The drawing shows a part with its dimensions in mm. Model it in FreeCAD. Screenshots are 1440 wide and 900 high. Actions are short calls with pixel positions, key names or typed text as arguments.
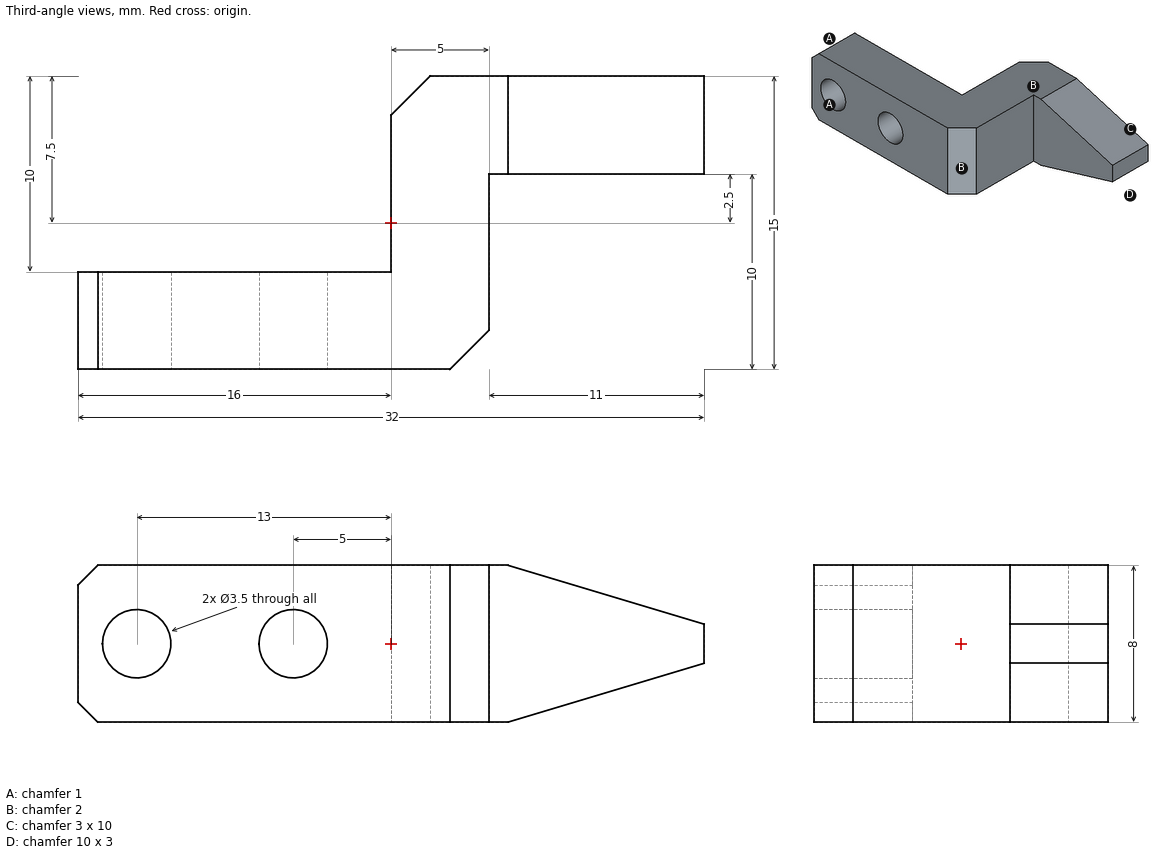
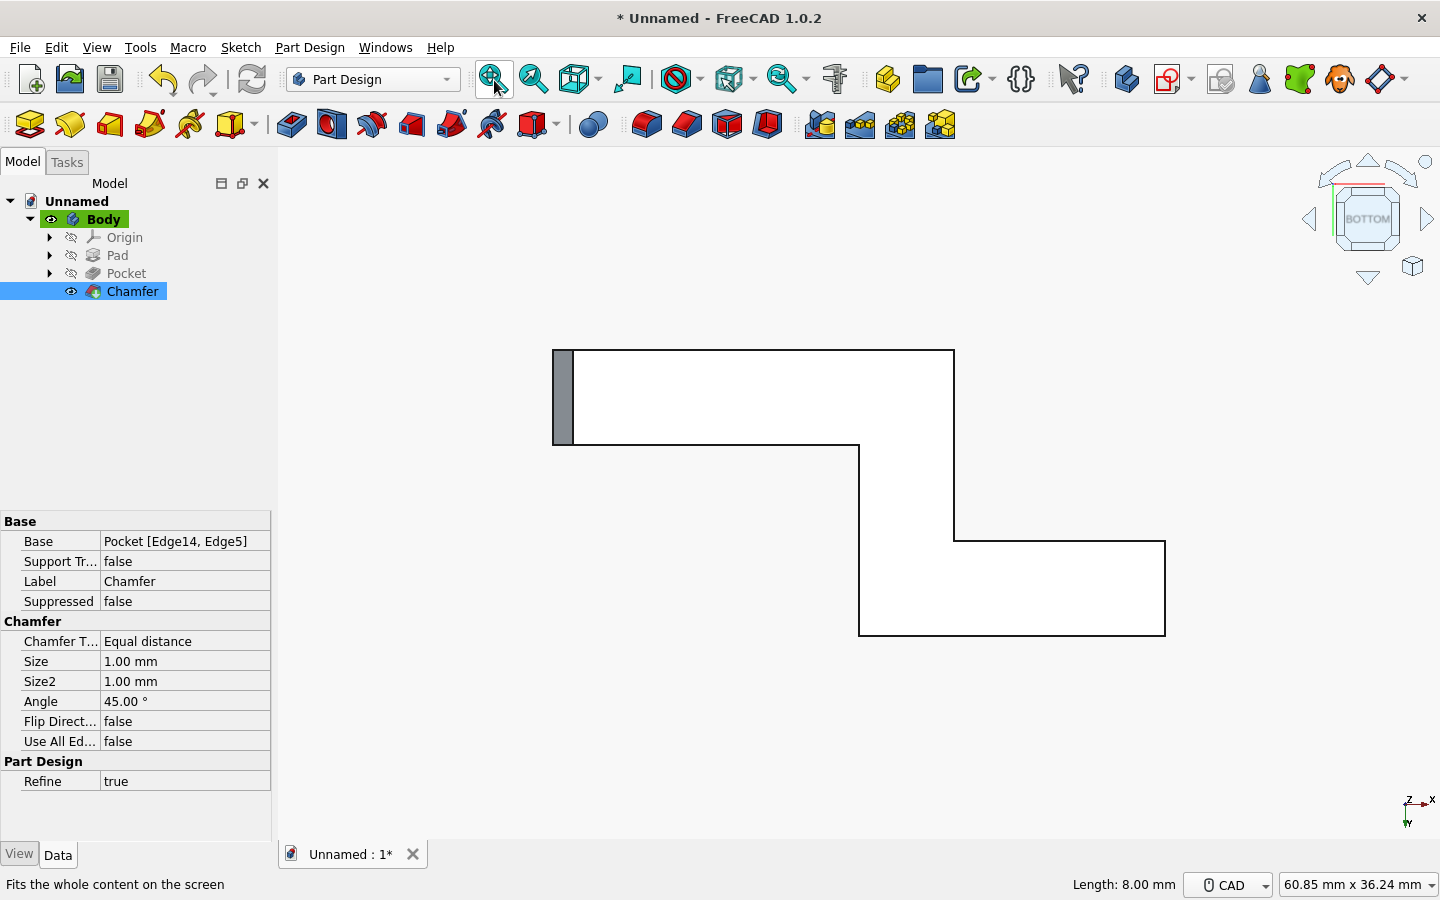
key(4)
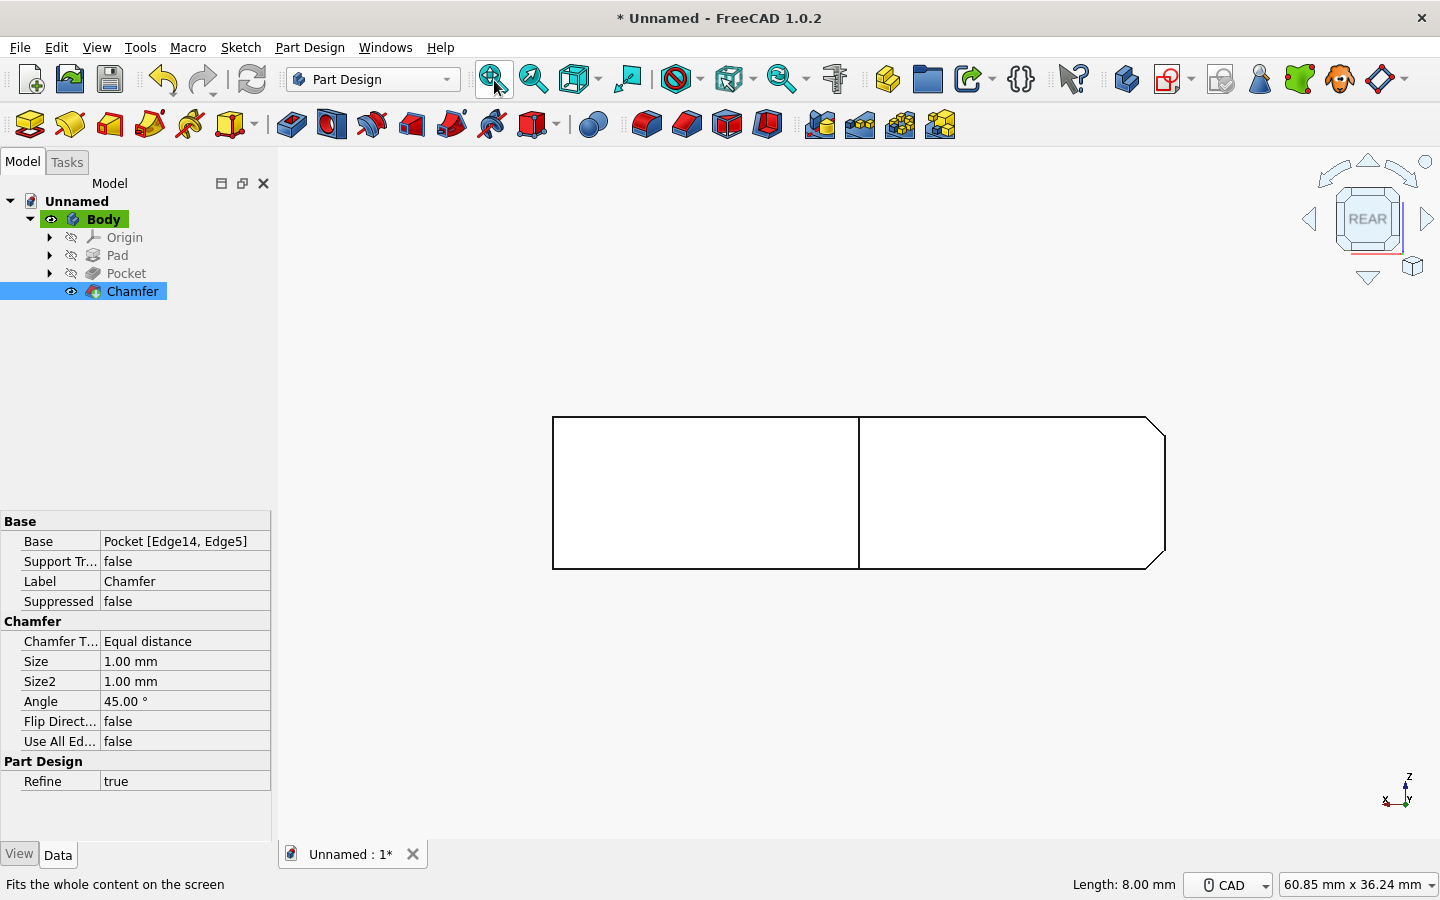
click(859, 492, ctrl)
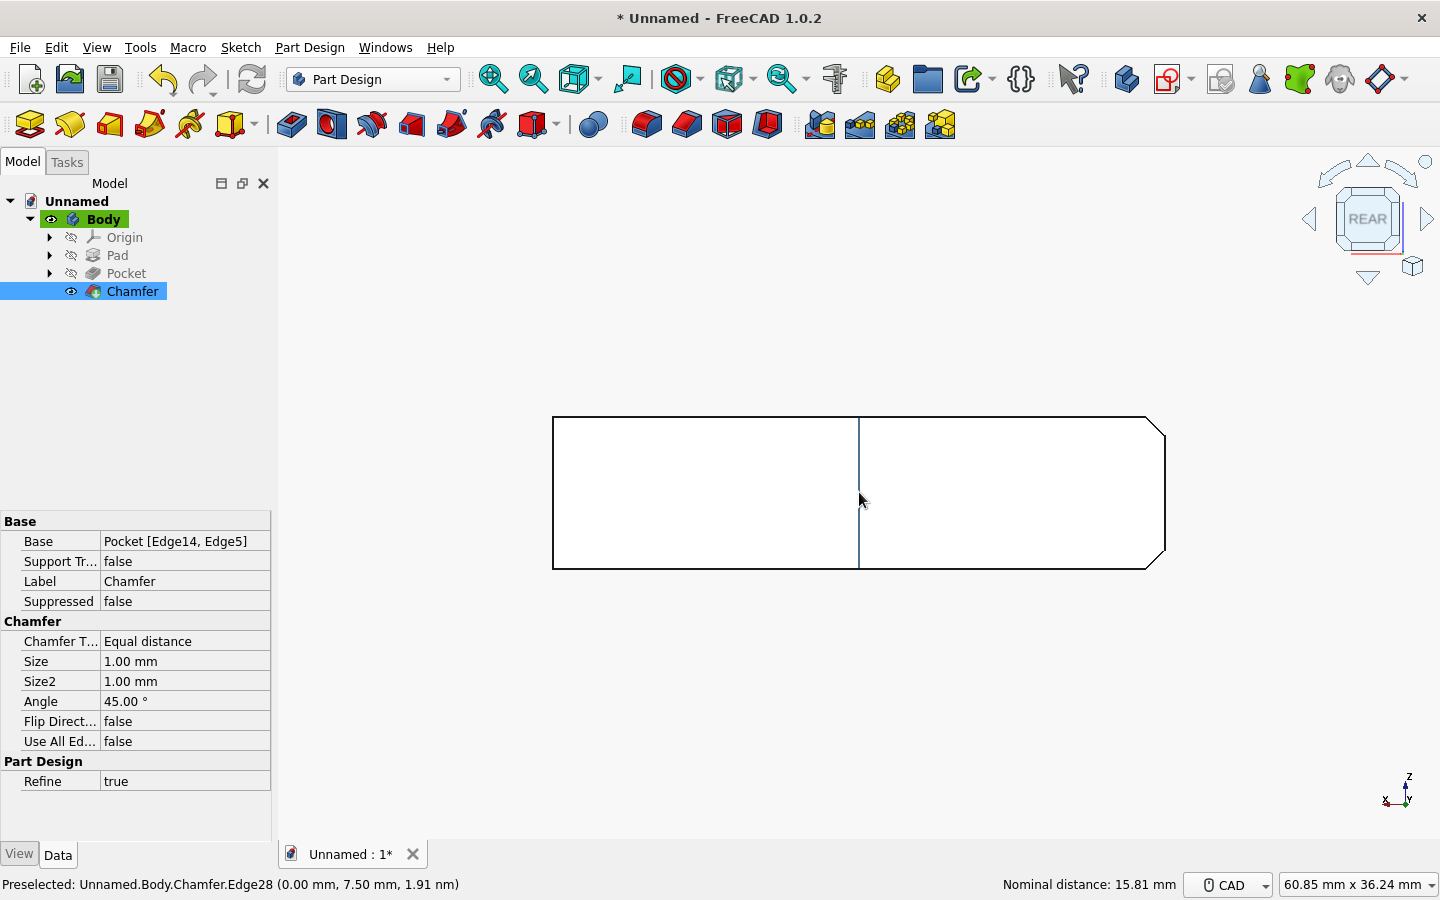
click(688, 124)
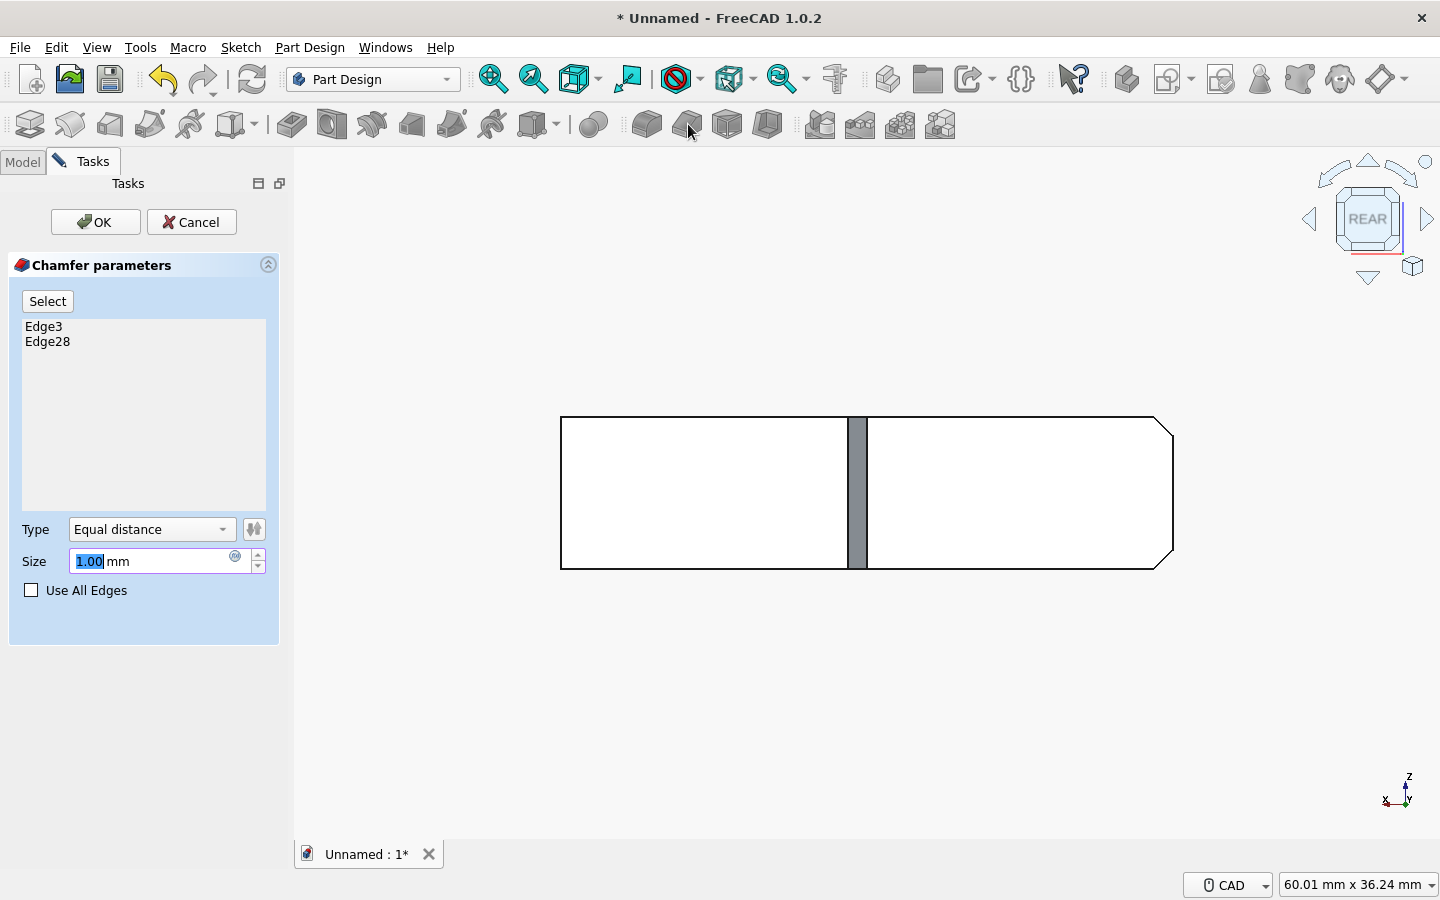
text(2)
key(Tab)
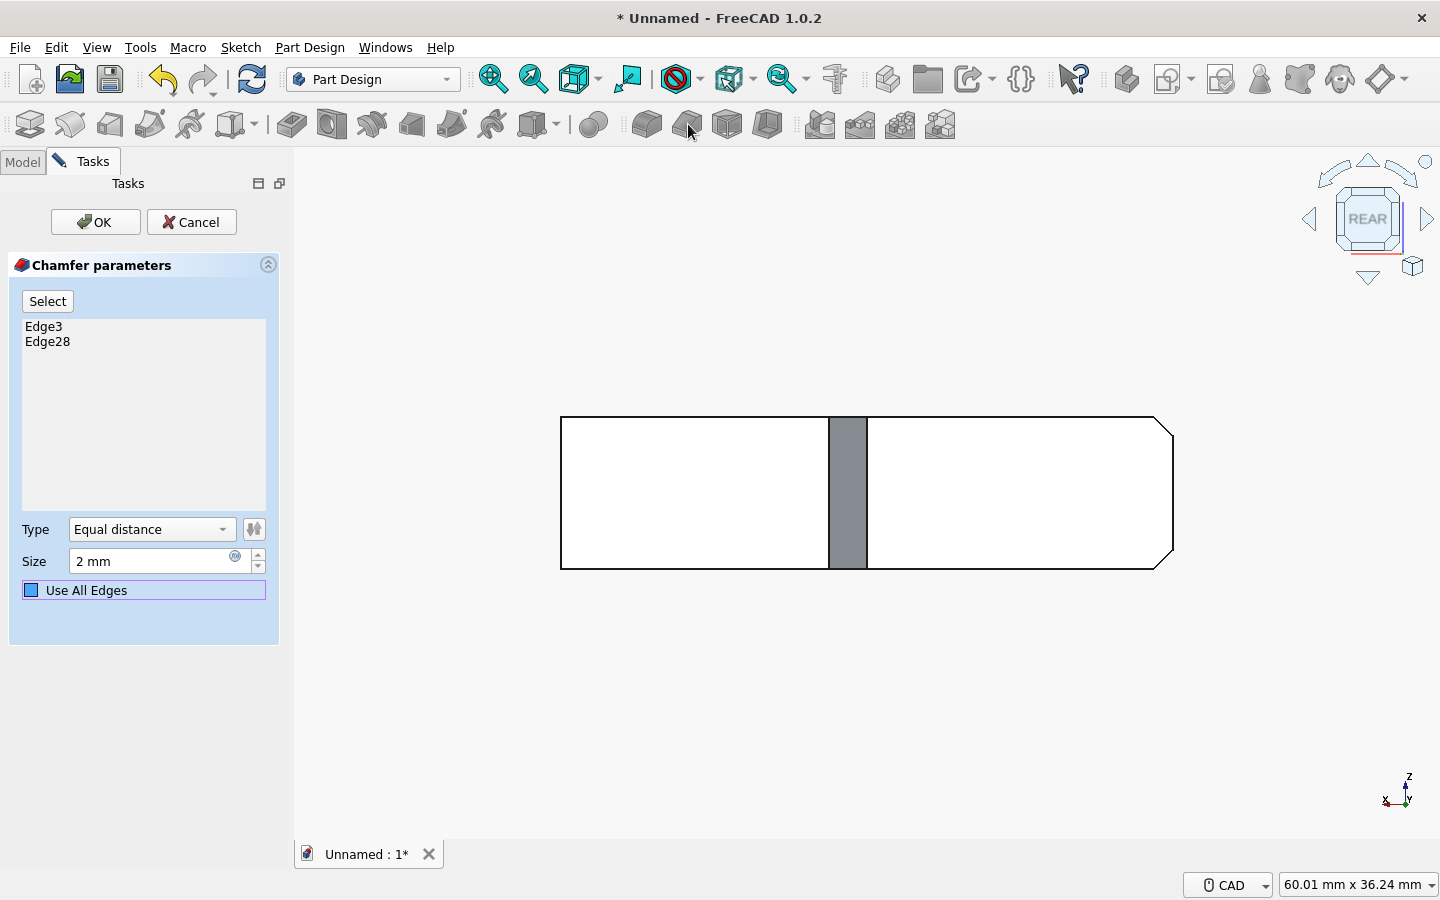
click(96, 222)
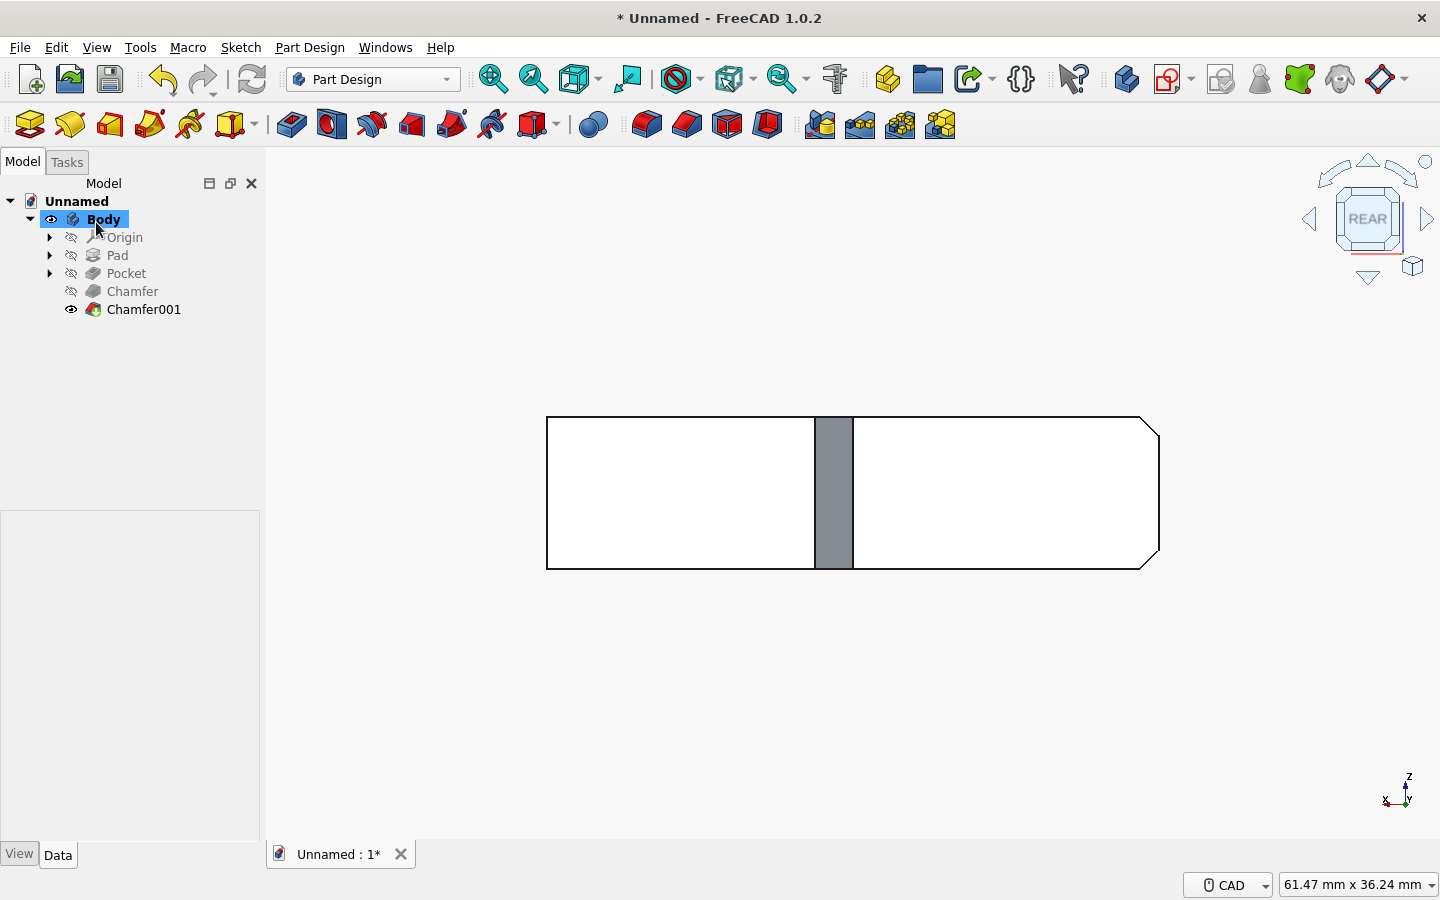
click(962, 492)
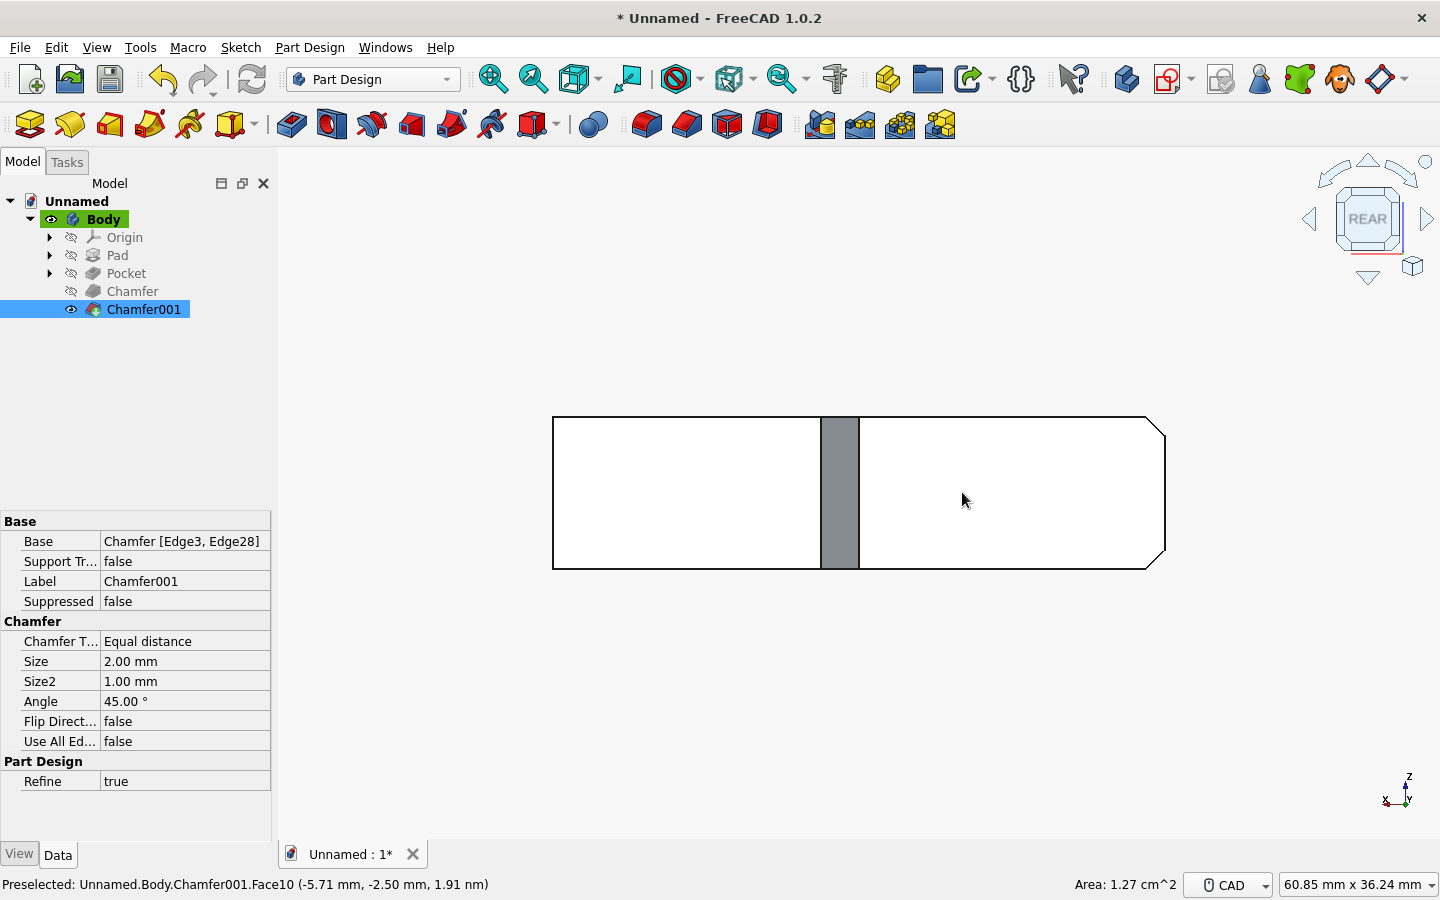
click(1168, 80)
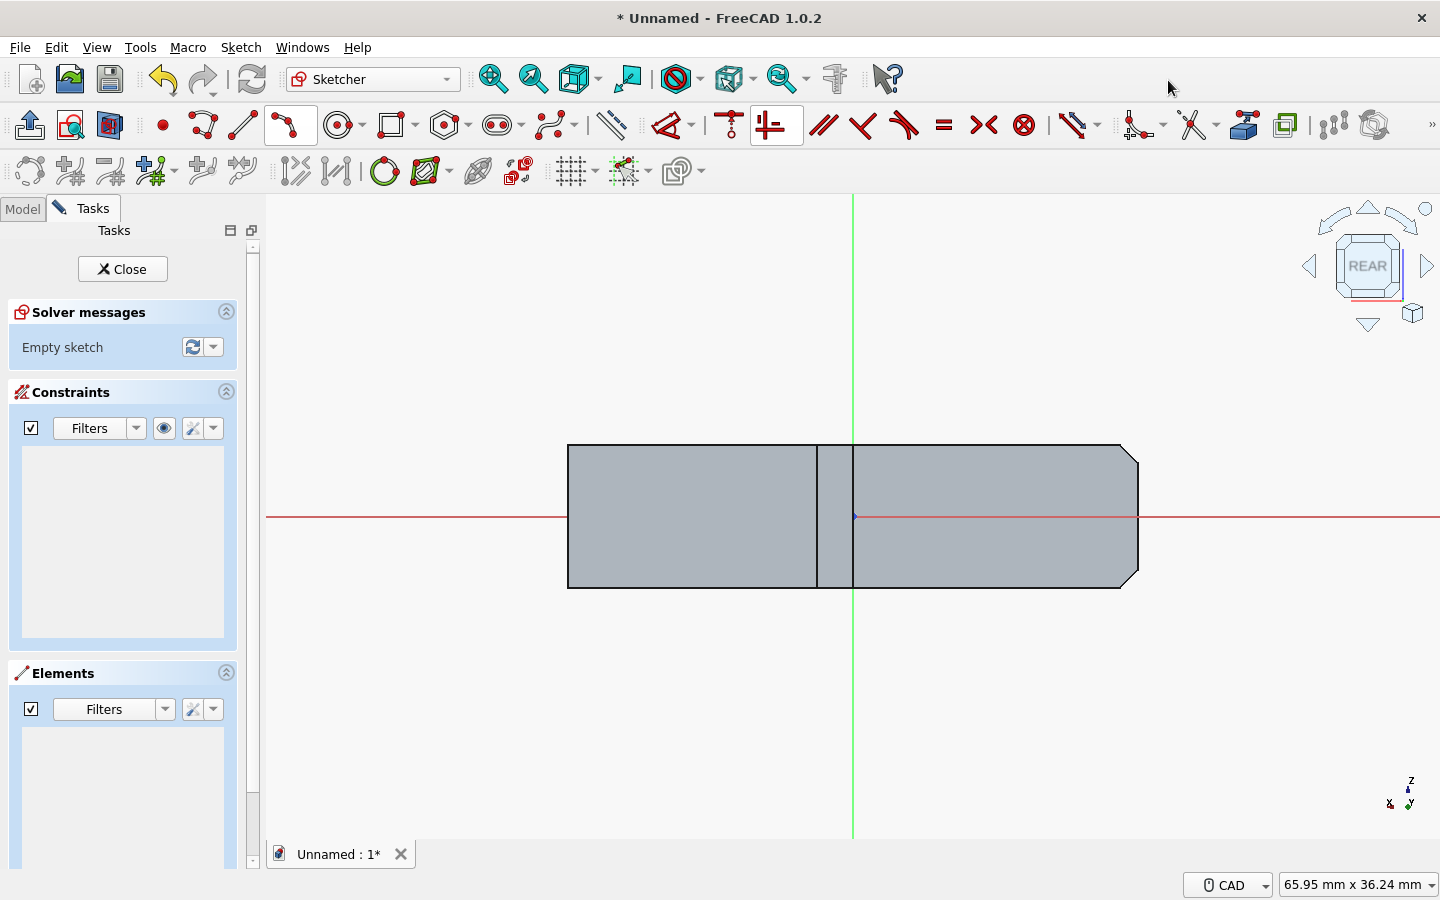
scroll(1101, 517, up, 5)